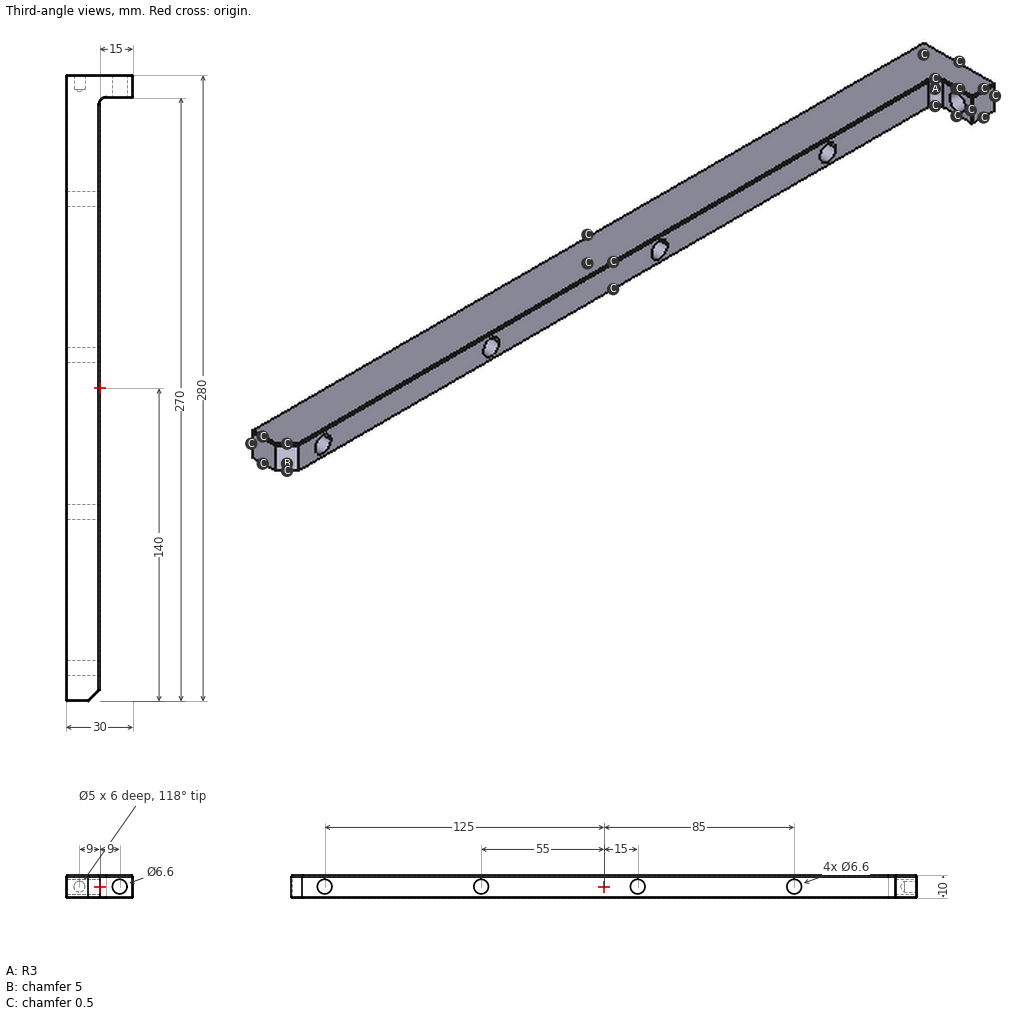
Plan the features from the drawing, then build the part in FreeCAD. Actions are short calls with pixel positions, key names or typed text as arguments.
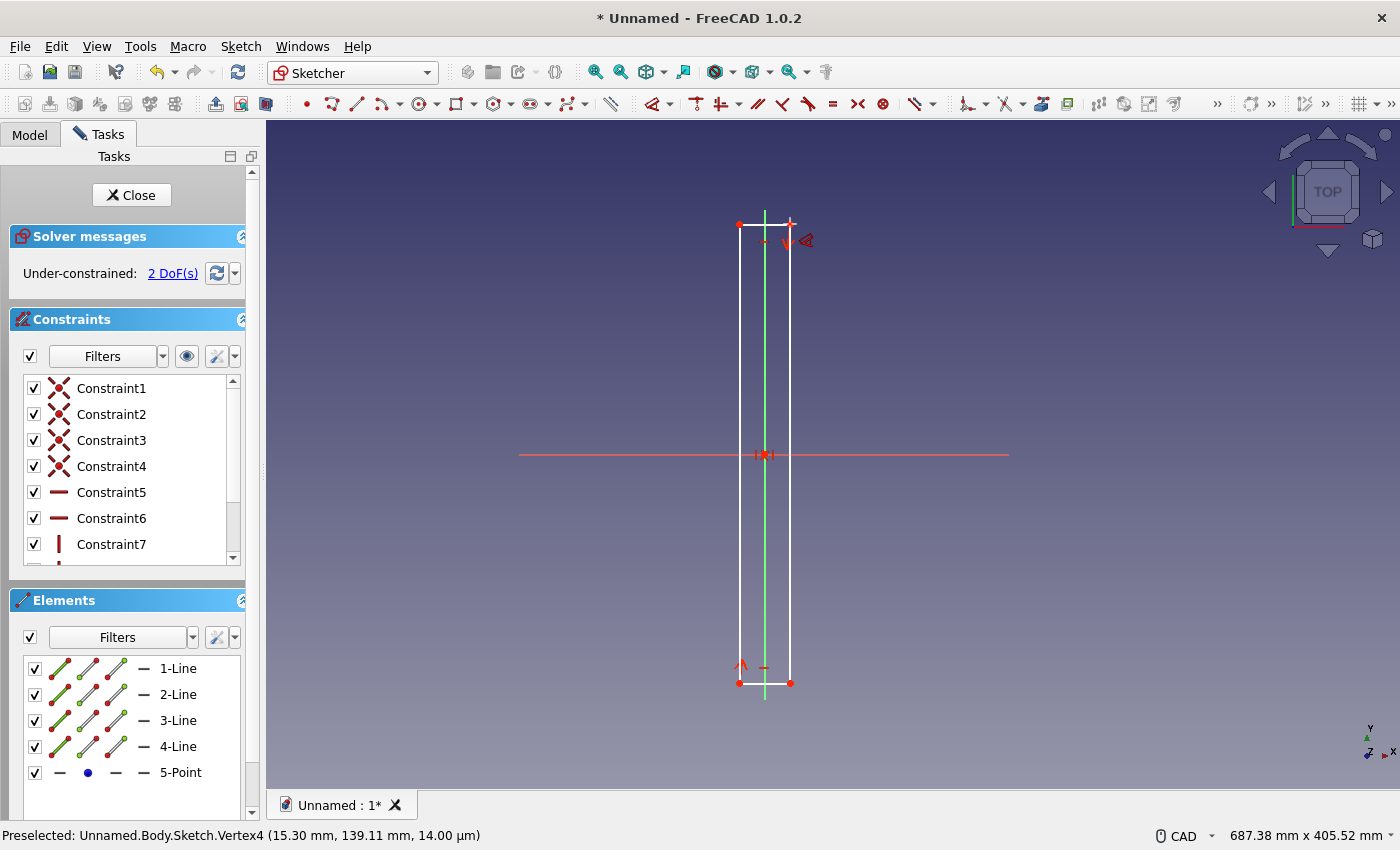
scroll(755, 684, up, 2)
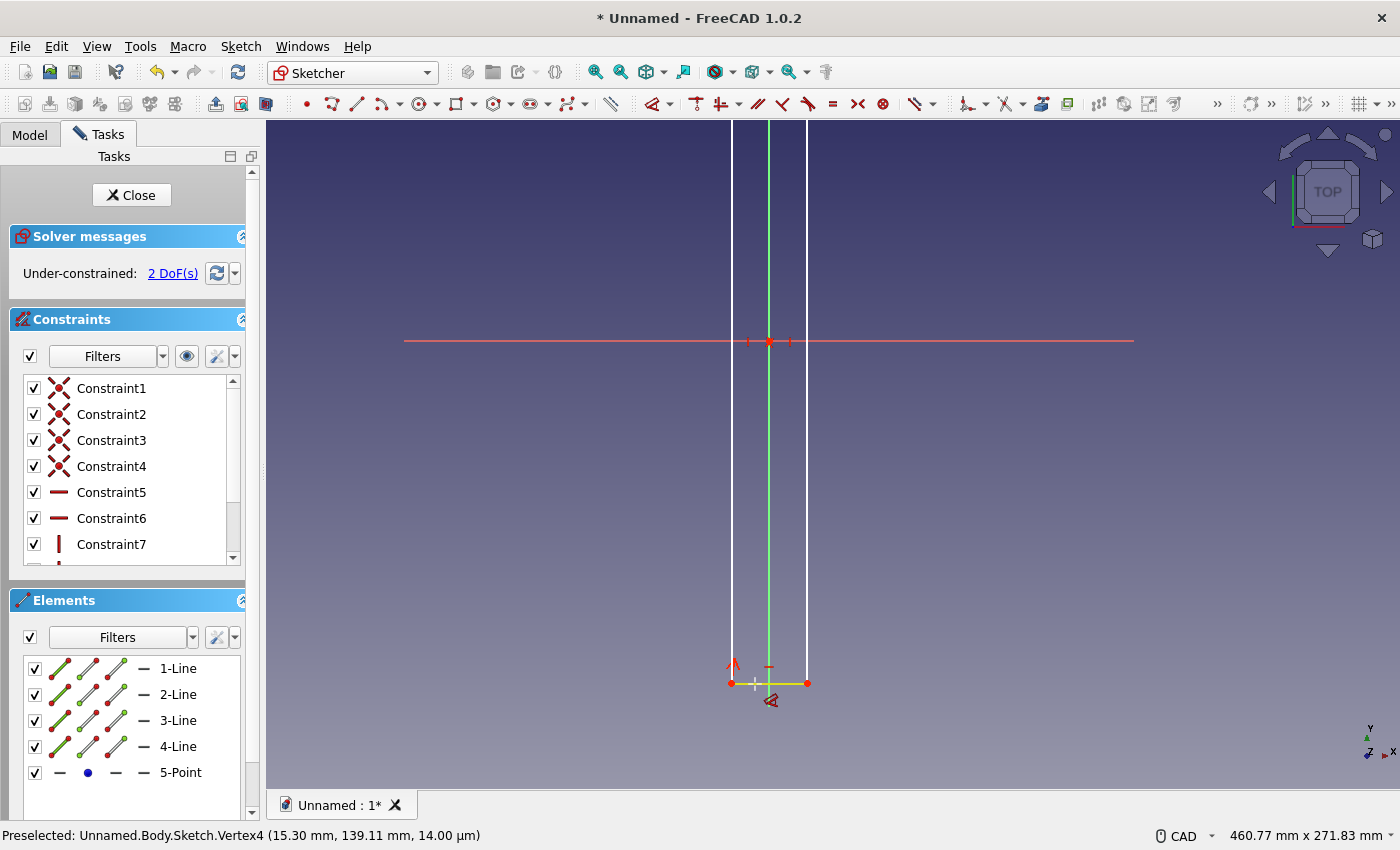
click(754, 684)
click(752, 718)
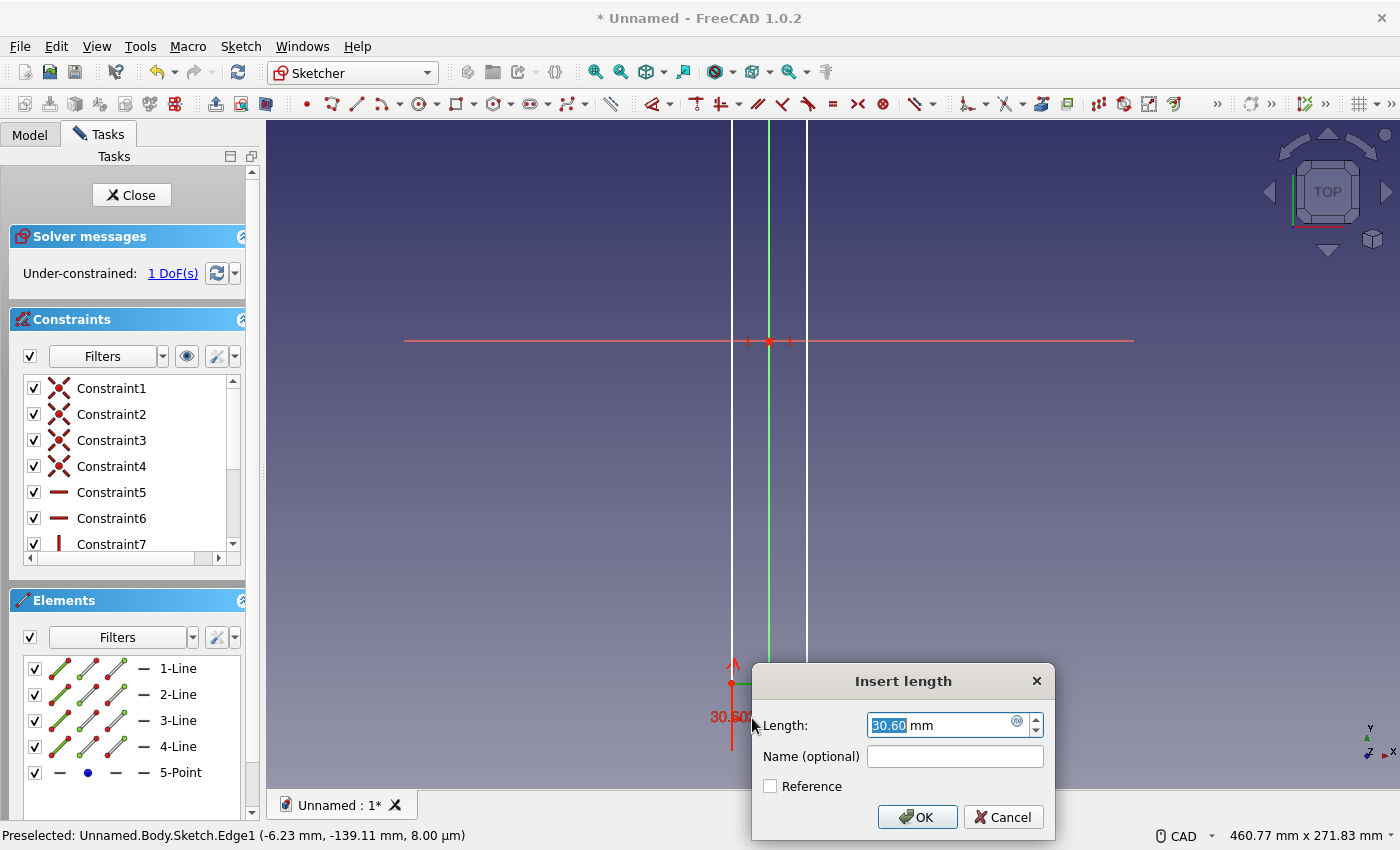
text(30)
key(Return)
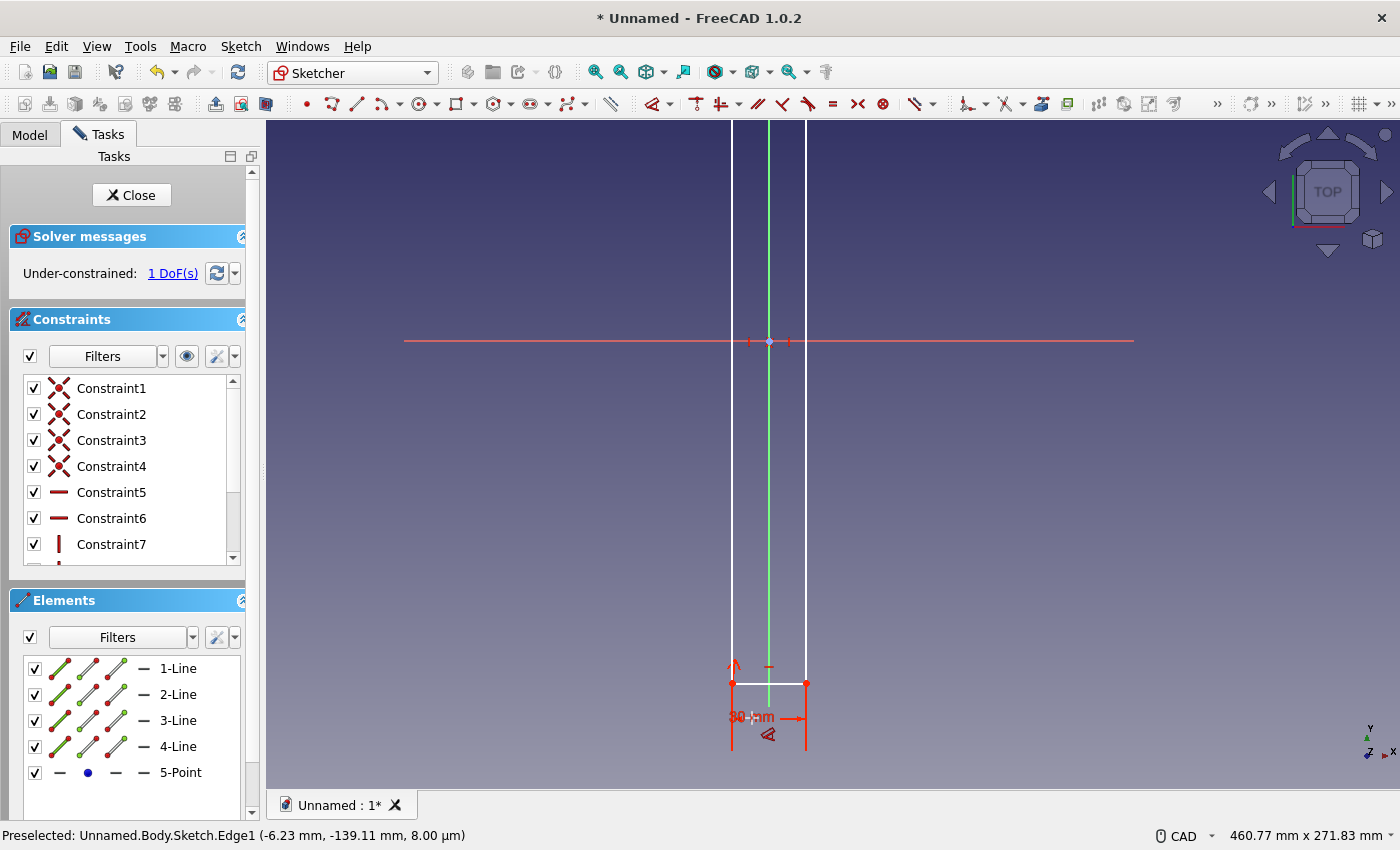
click(806, 478)
click(840, 416)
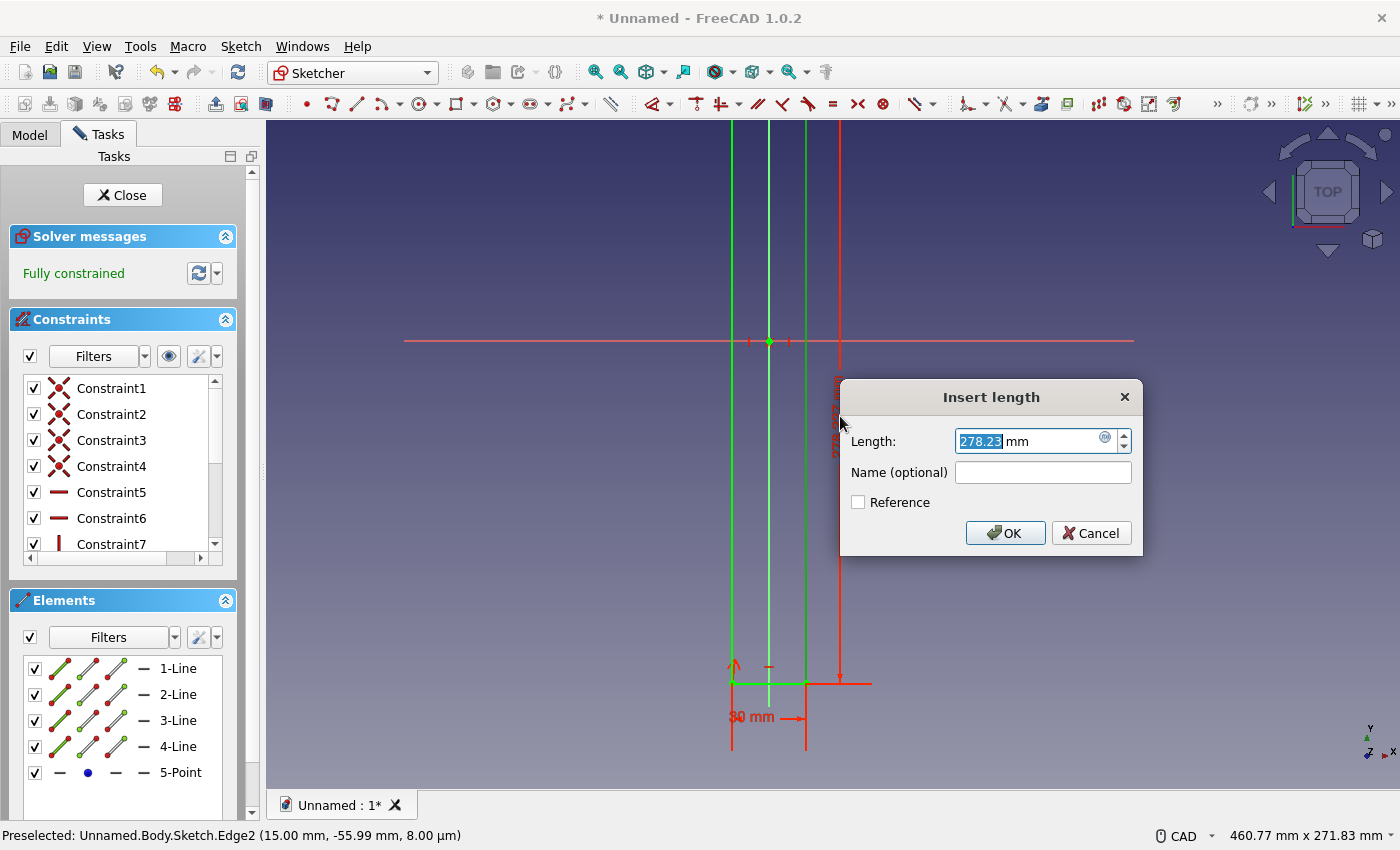
text(280)
key(Return)
key(Escape)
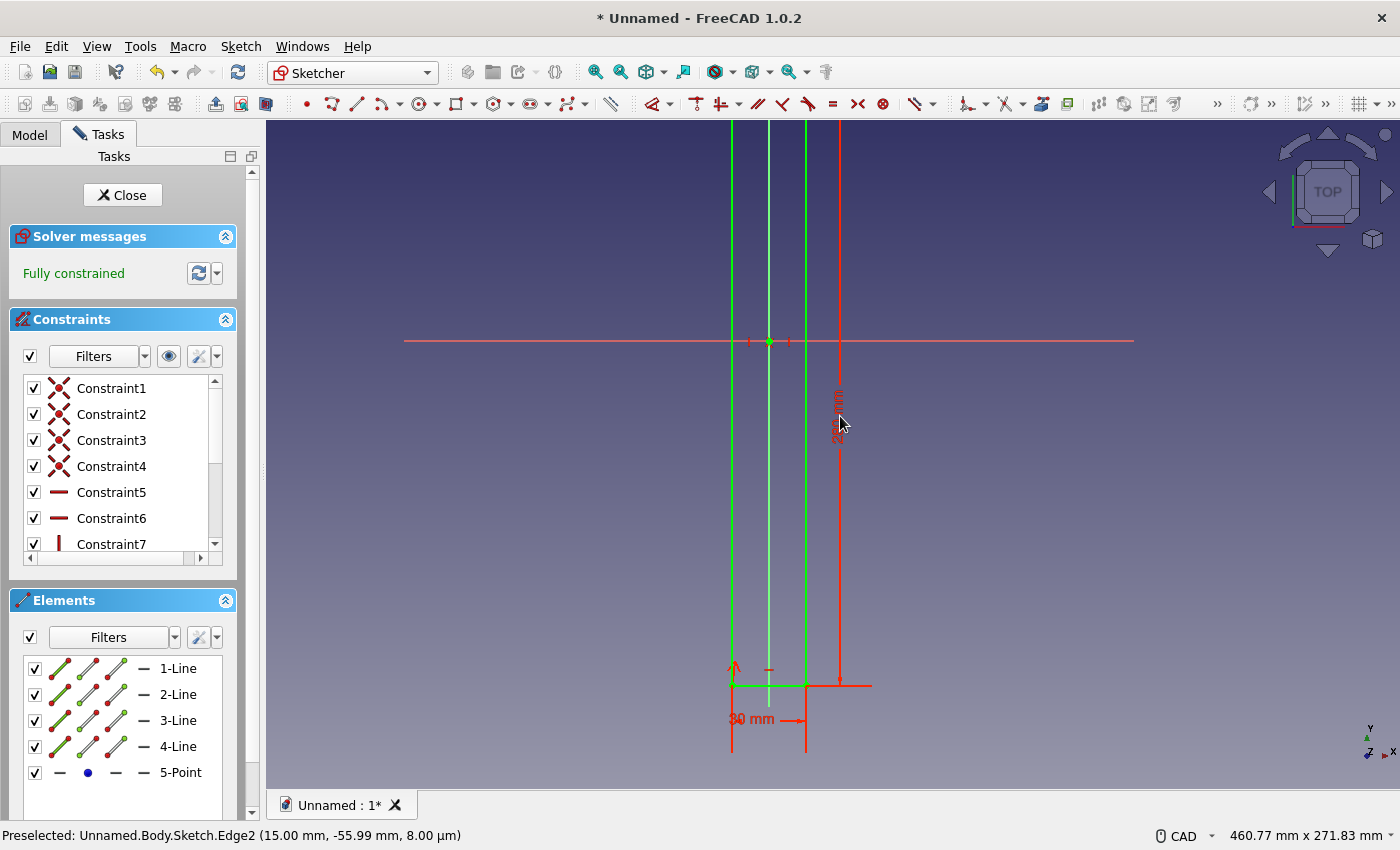
click(123, 195)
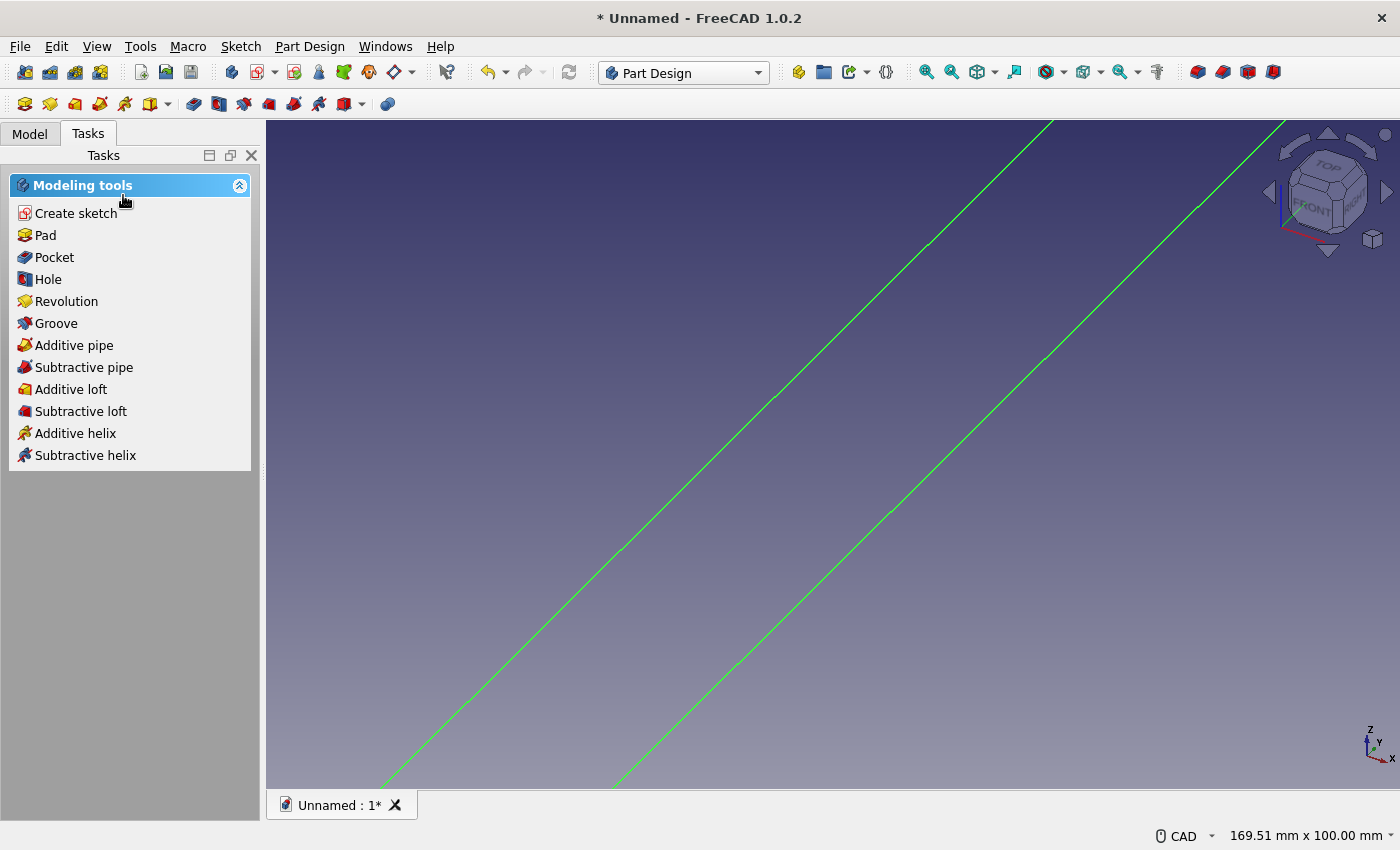
click(25, 104)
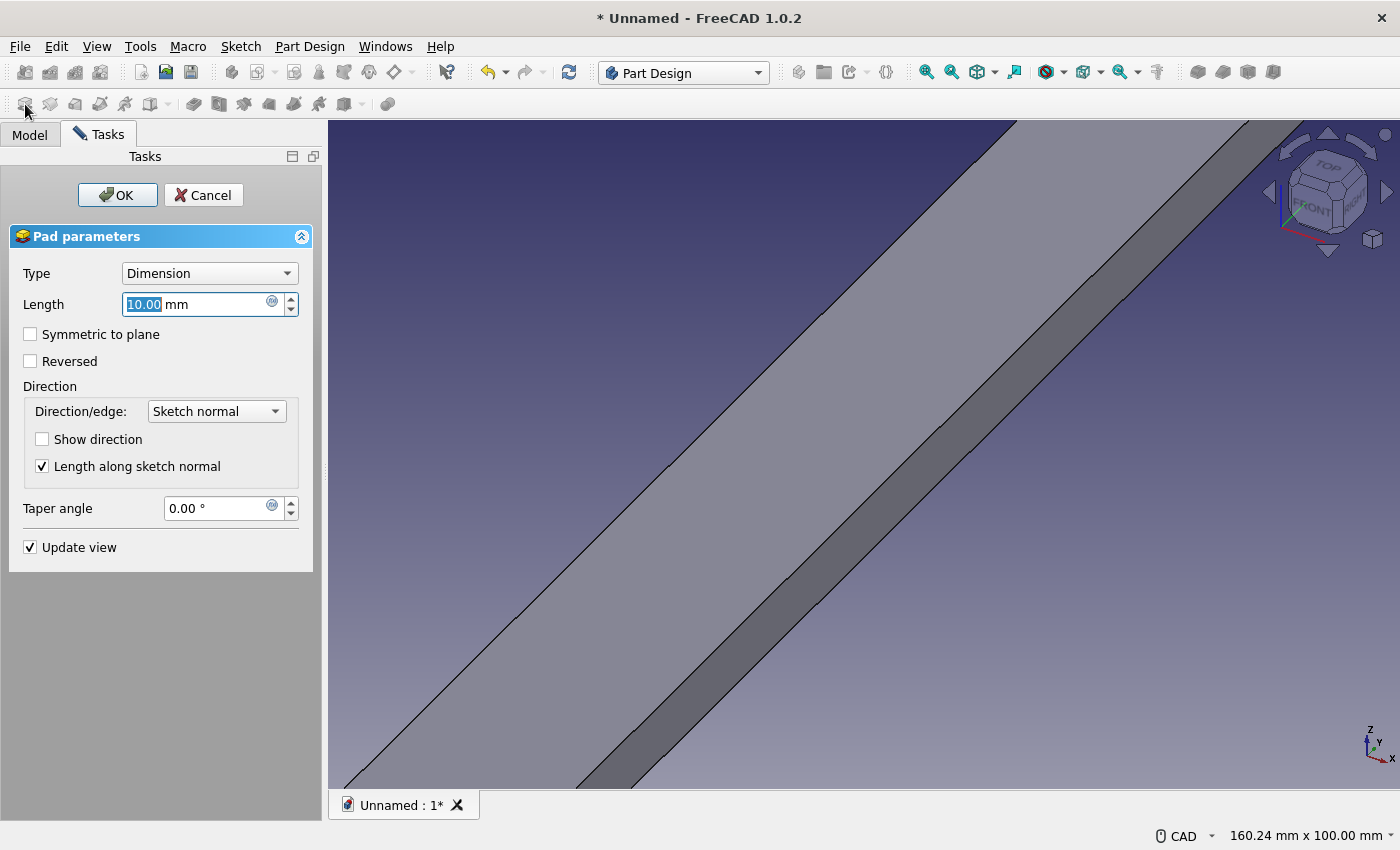
text(10)
key(Tab)